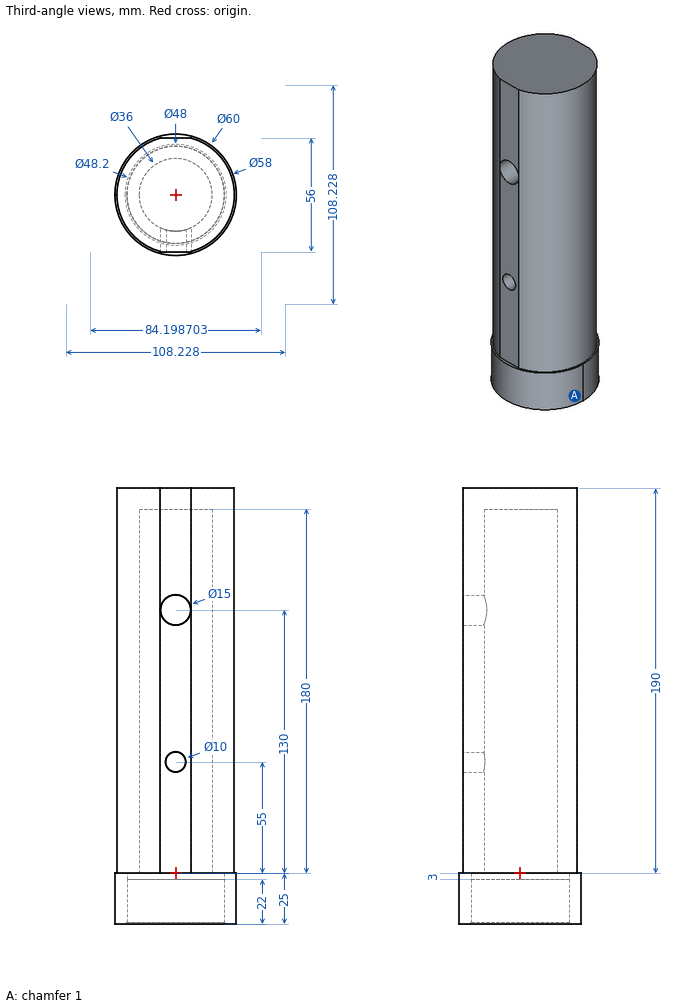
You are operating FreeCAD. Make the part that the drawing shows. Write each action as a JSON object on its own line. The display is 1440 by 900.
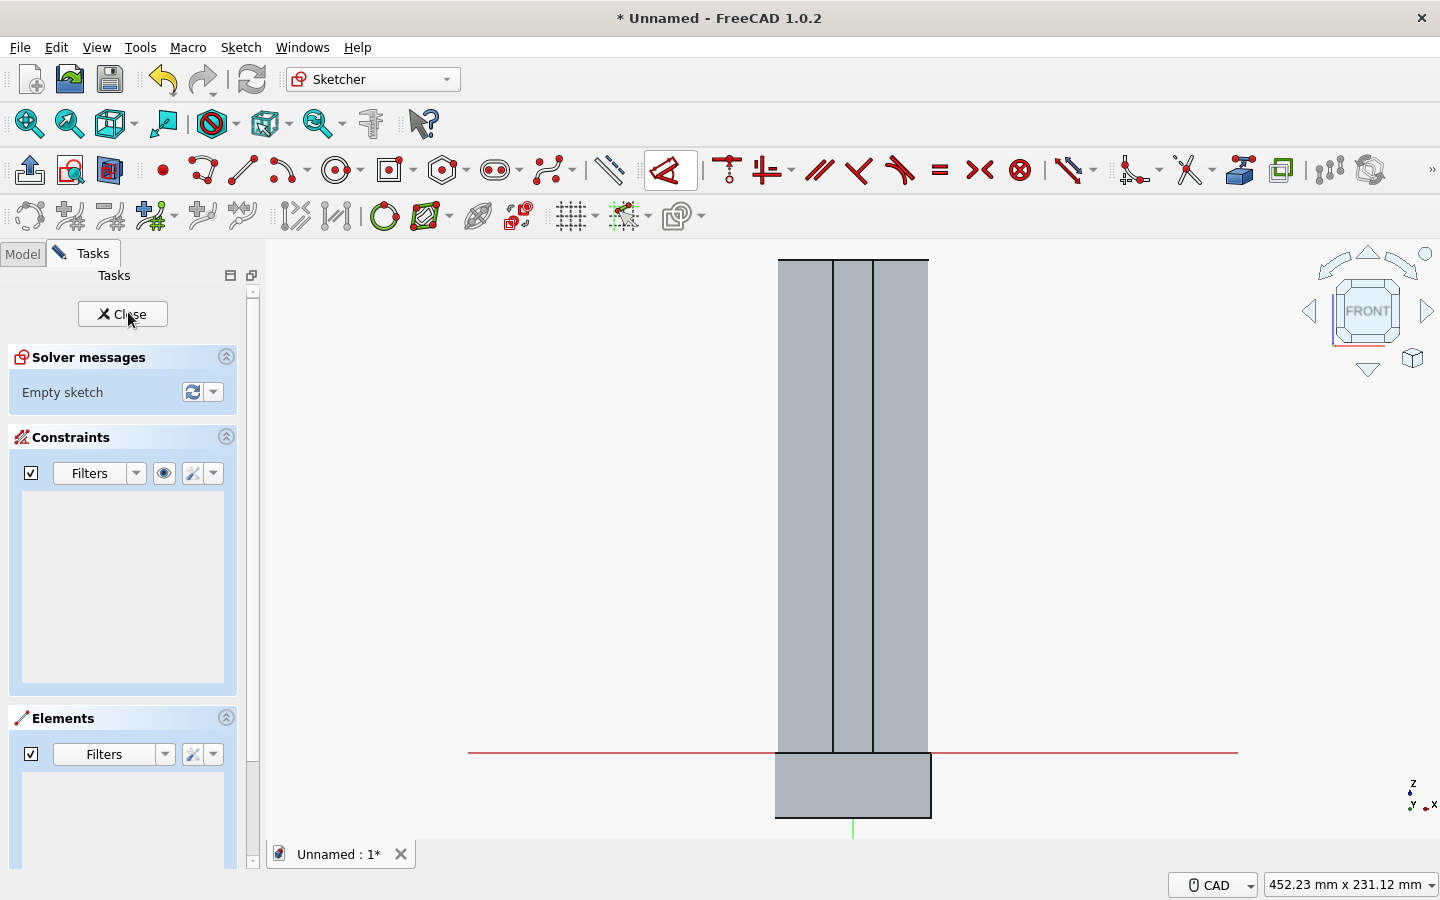
{"action": "left_click", "coordinate": [110, 170]}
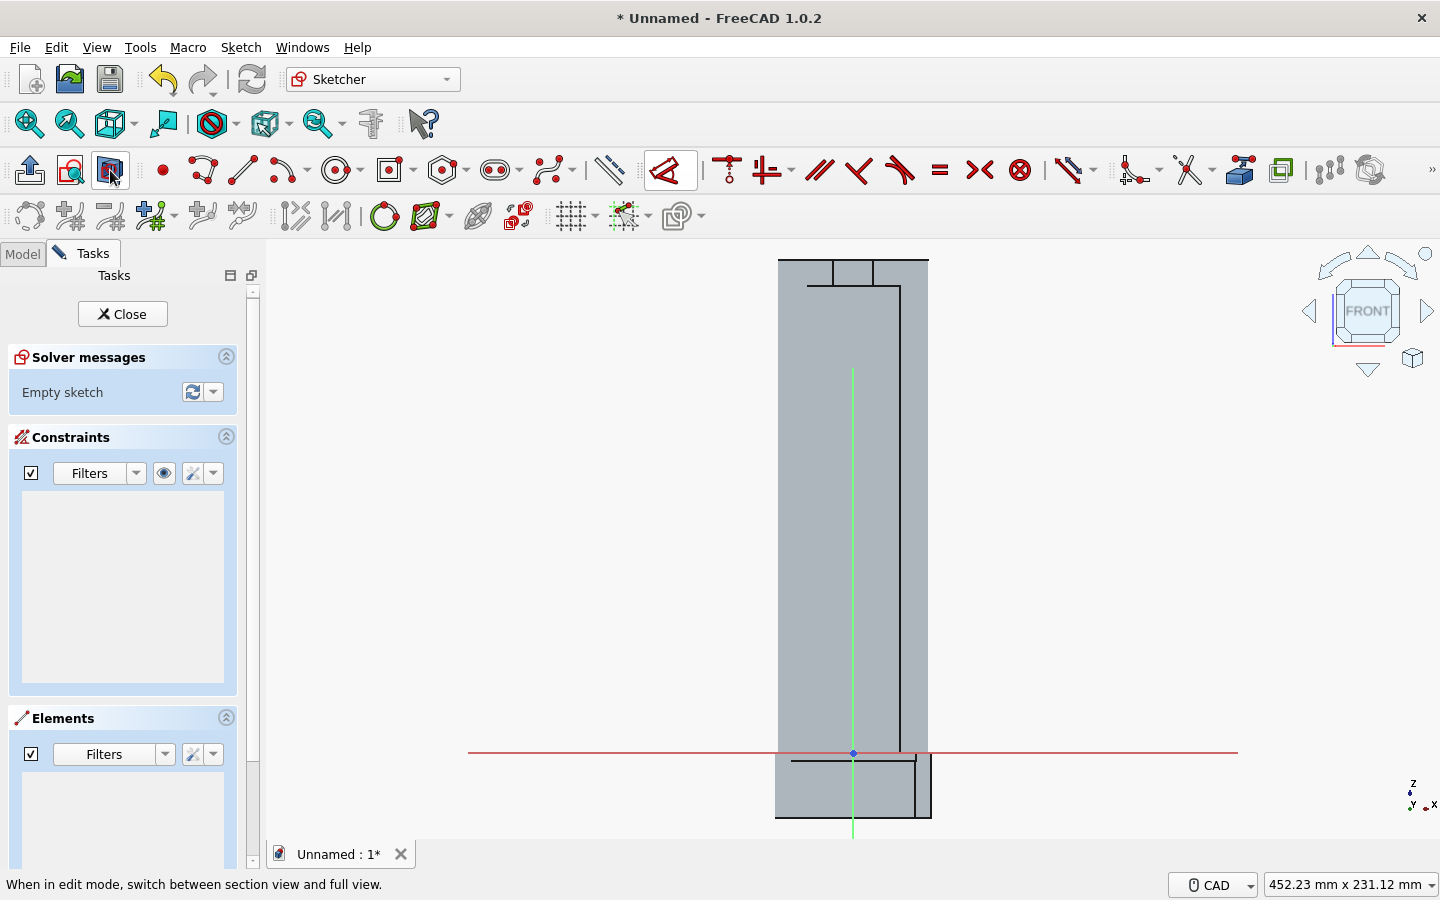
{"action": "left_click", "coordinate": [336, 170]}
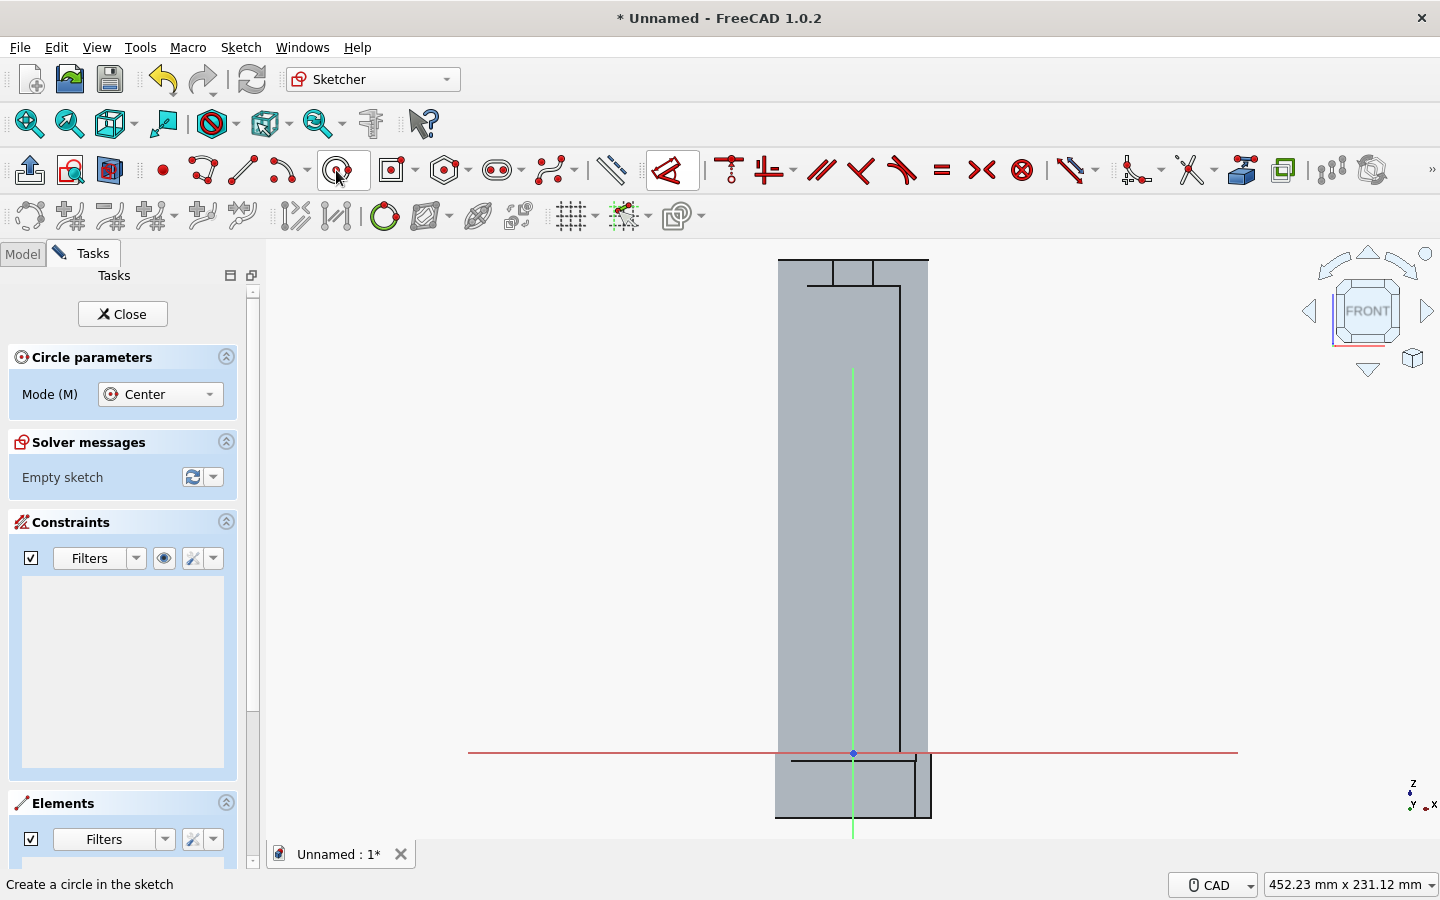
{"action": "scroll", "coordinate": [853, 610], "scroll_direction": "up", "scroll_amount": 3}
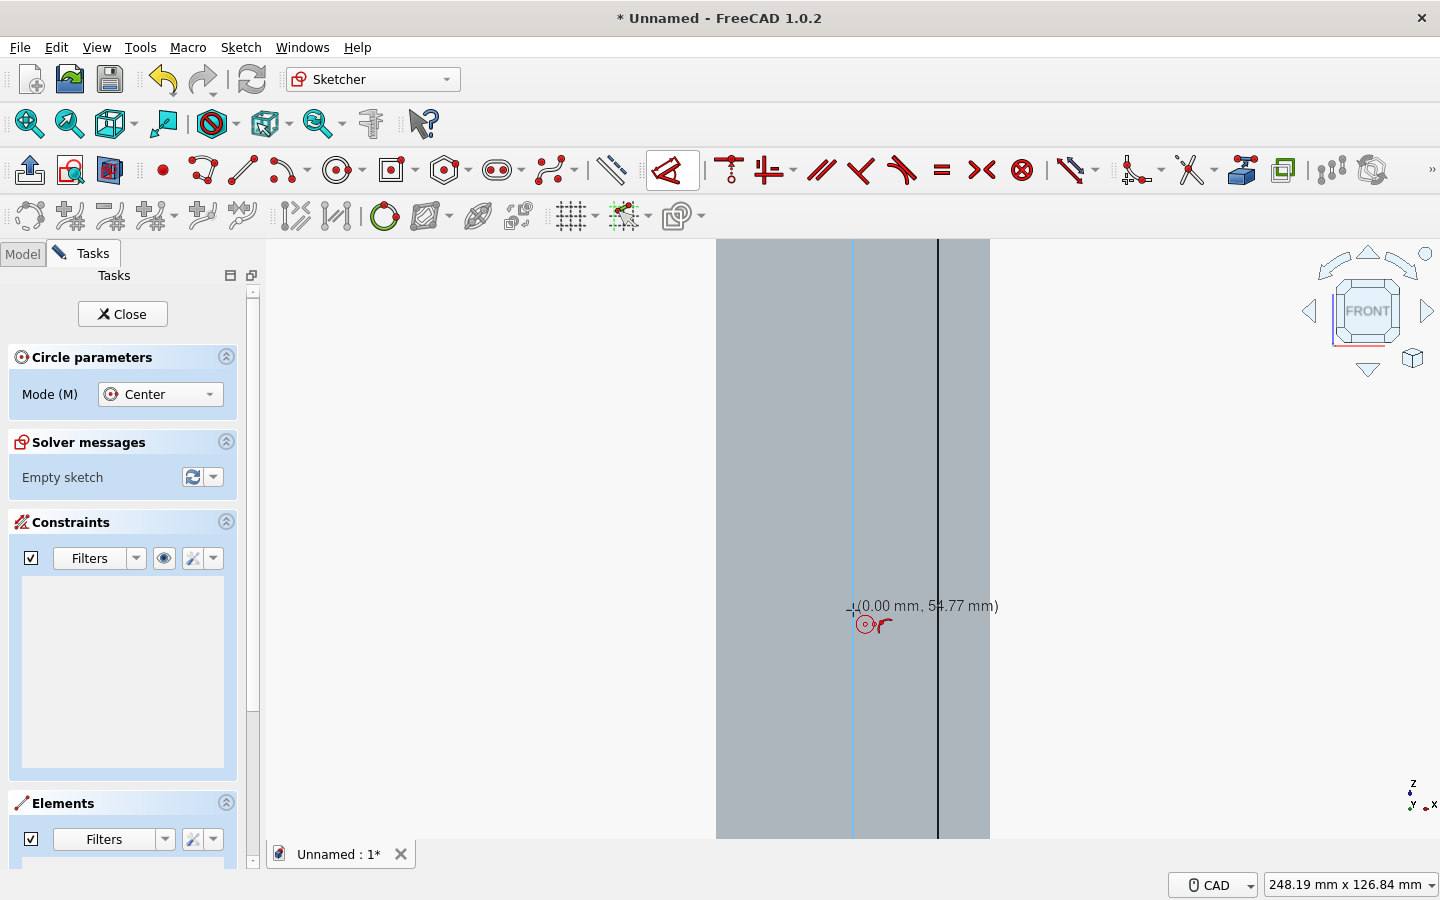
{"action": "left_click", "coordinate": [853, 610]}
{"action": "left_click", "coordinate": [869, 593]}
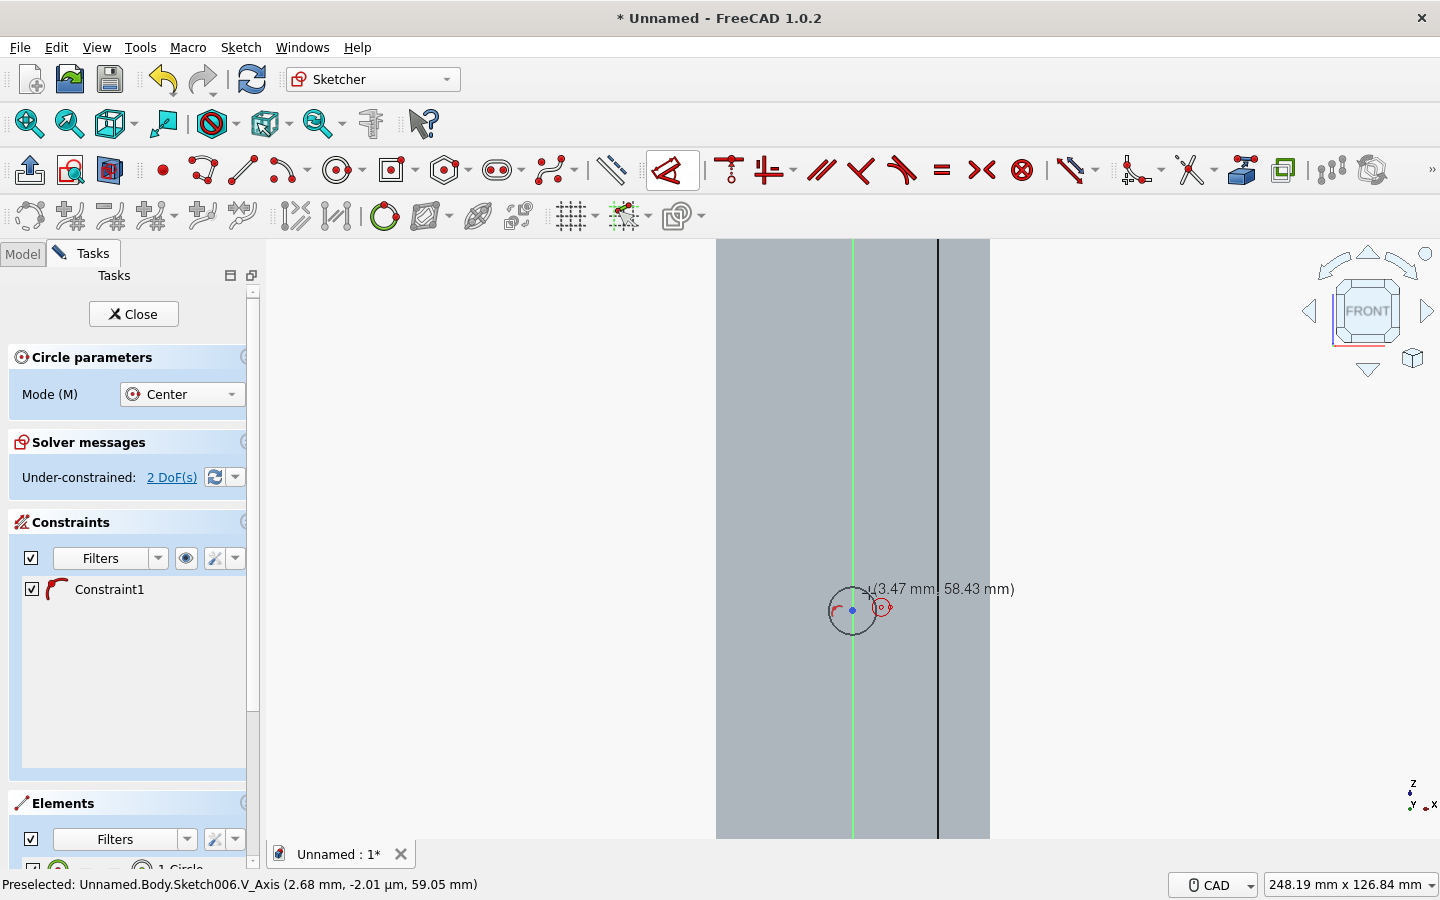
{"action": "scroll", "coordinate": [702, 532], "scroll_direction": "down", "scroll_amount": 3}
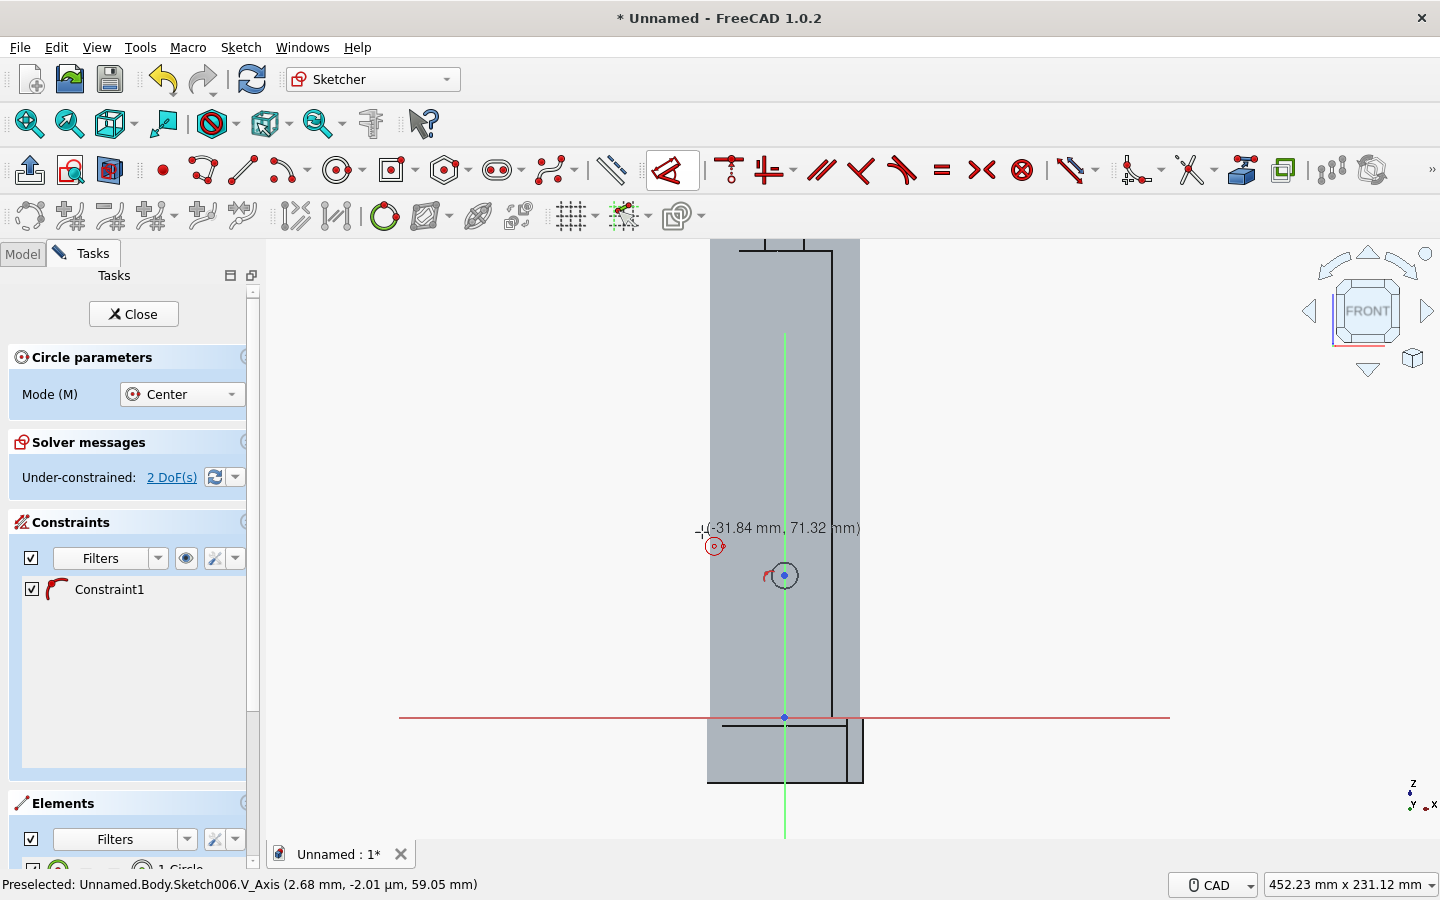
{"action": "left_click", "coordinate": [785, 380]}
{"action": "left_click", "coordinate": [803, 374]}
{"action": "key", "text": "Escape"}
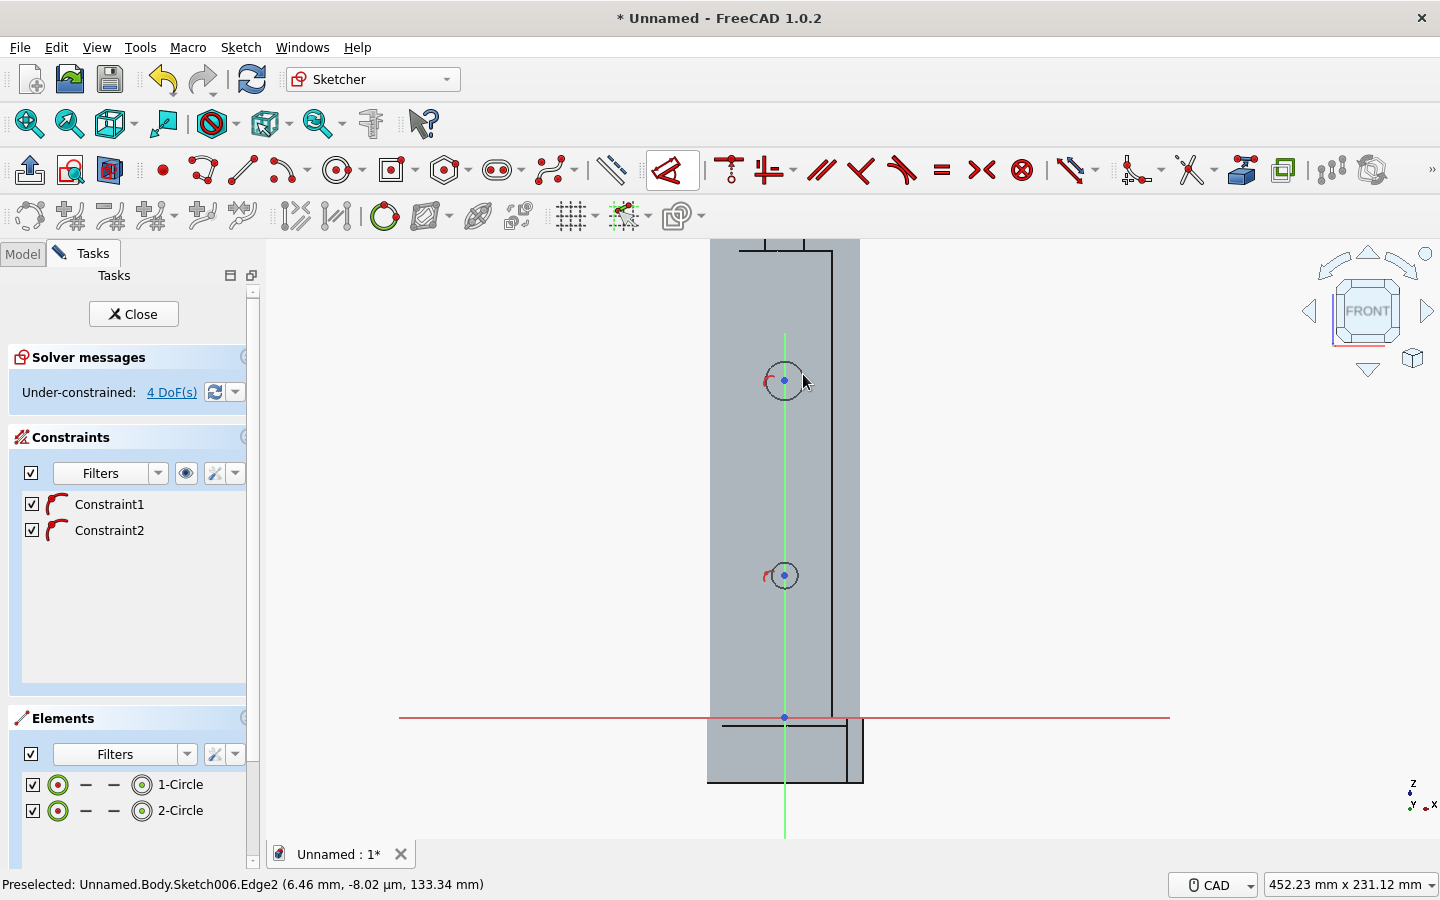
{"action": "scroll", "coordinate": [794, 566], "scroll_direction": "up", "scroll_amount": 3}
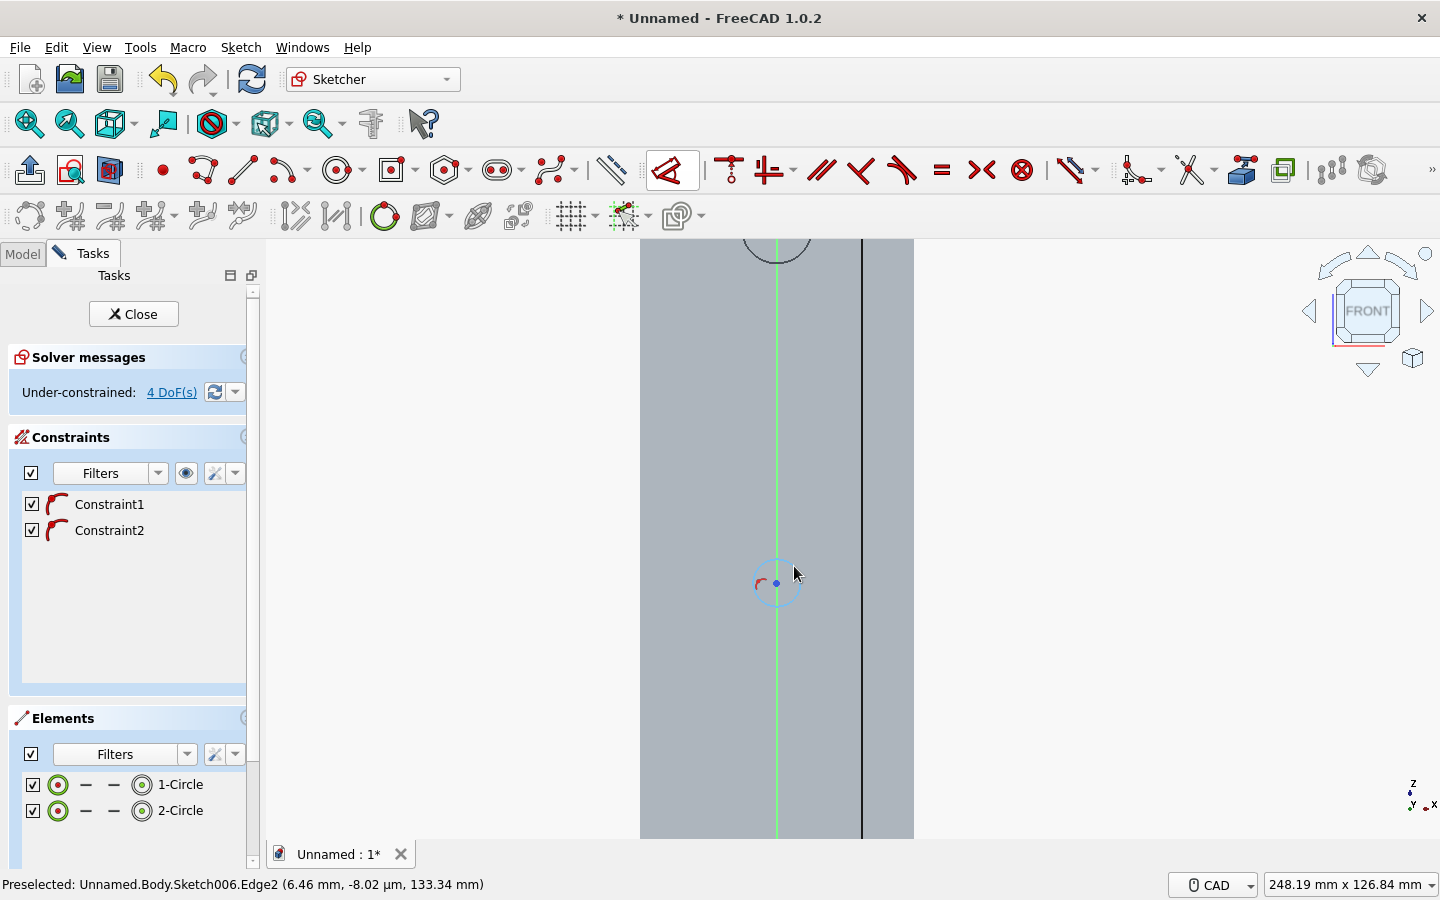
{"action": "left_click", "coordinate": [794, 566]}